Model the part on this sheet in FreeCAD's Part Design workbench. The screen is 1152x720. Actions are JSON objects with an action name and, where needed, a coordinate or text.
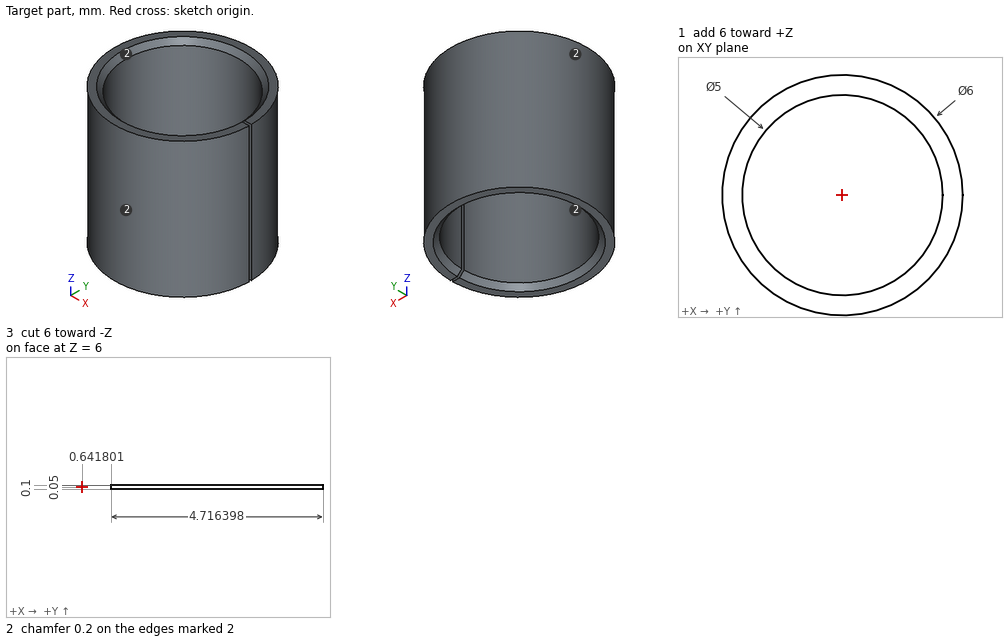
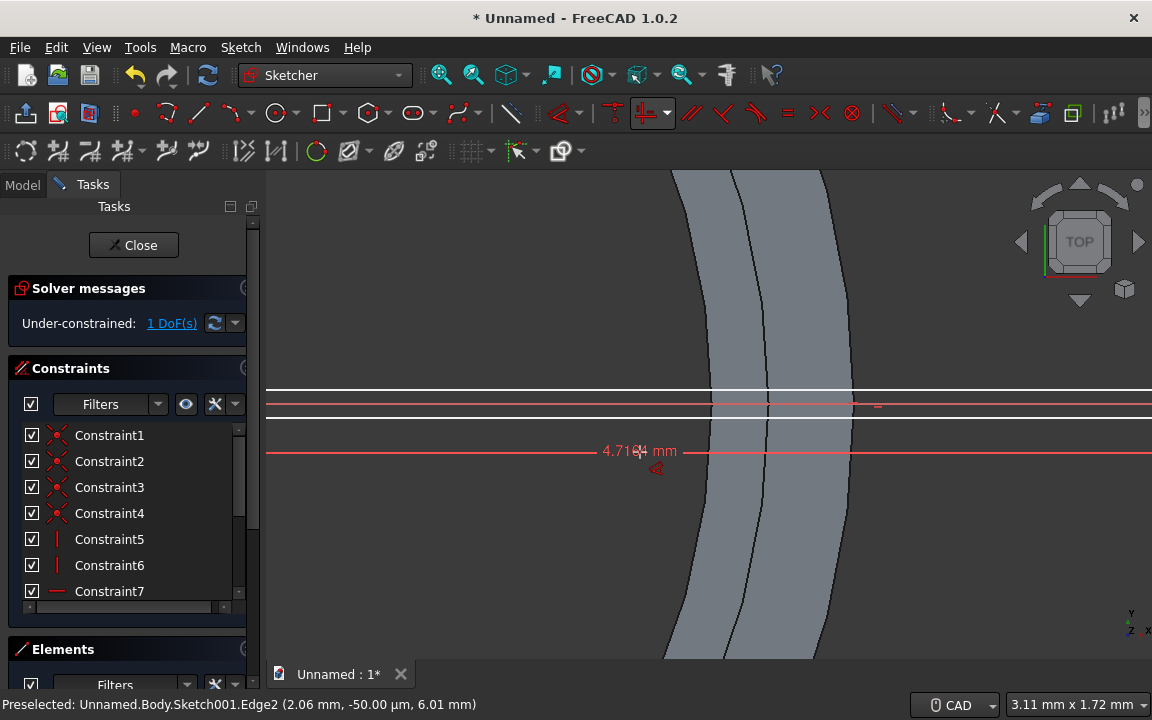
{"action": "scroll", "coordinate": [588, 419], "scroll_direction": "down", "scroll_amount": 6}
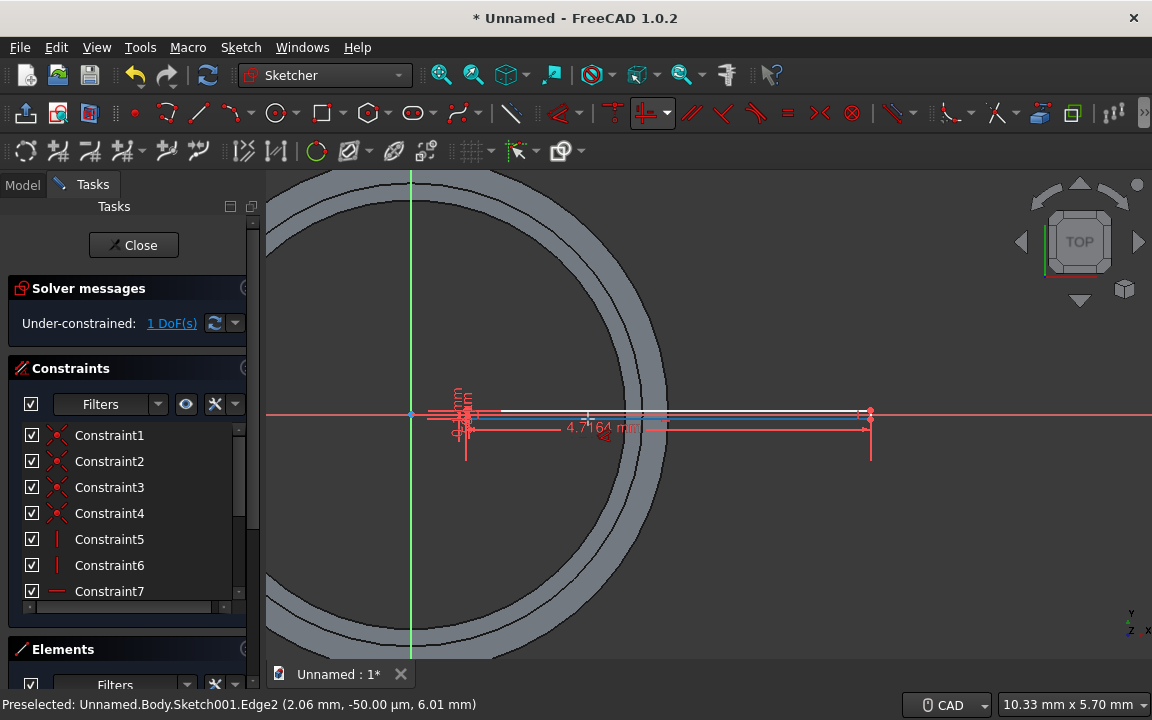
{"action": "scroll", "coordinate": [466, 411], "scroll_direction": "up", "scroll_amount": 2}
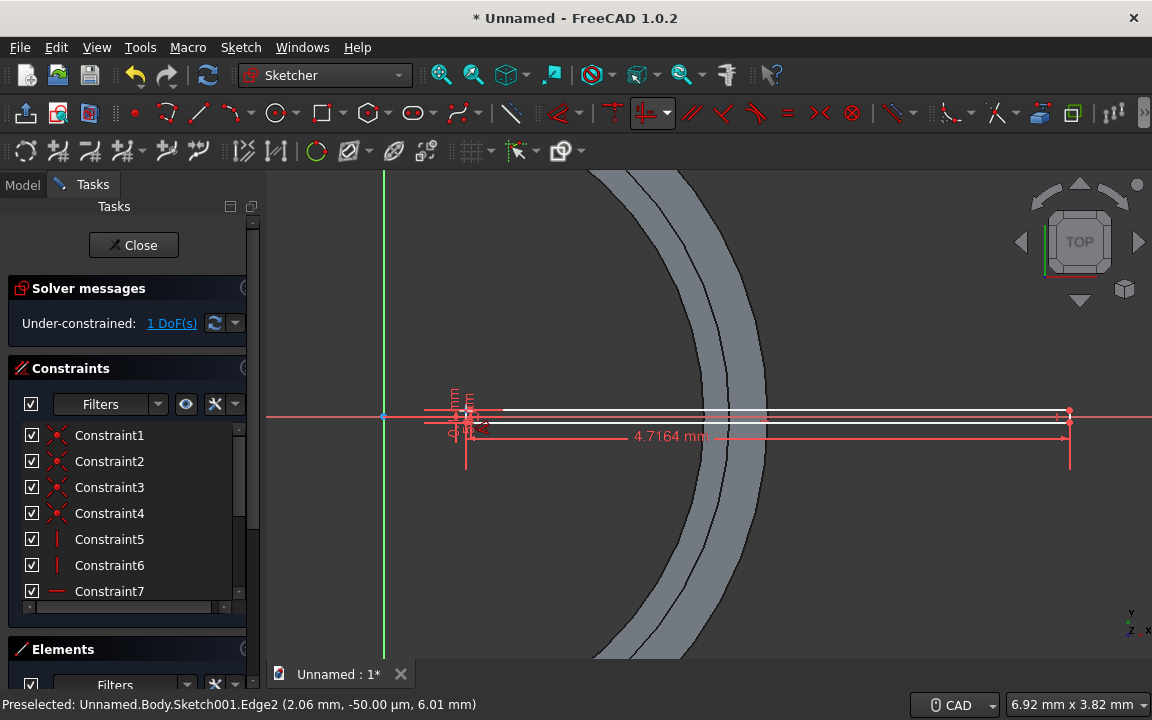
{"action": "left_click", "coordinate": [466, 410]}
{"action": "left_click", "coordinate": [425, 376]}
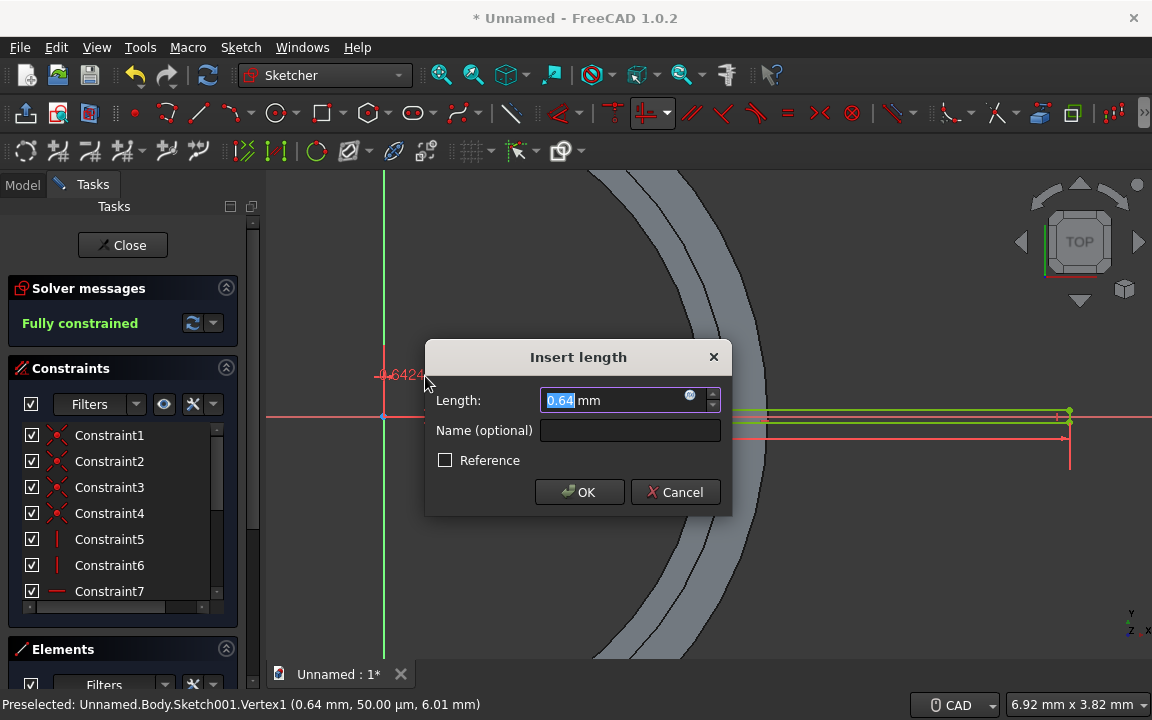
{"action": "type", "text": "0.641801"}
{"action": "key", "text": "Return"}
{"action": "key", "text": "Escape"}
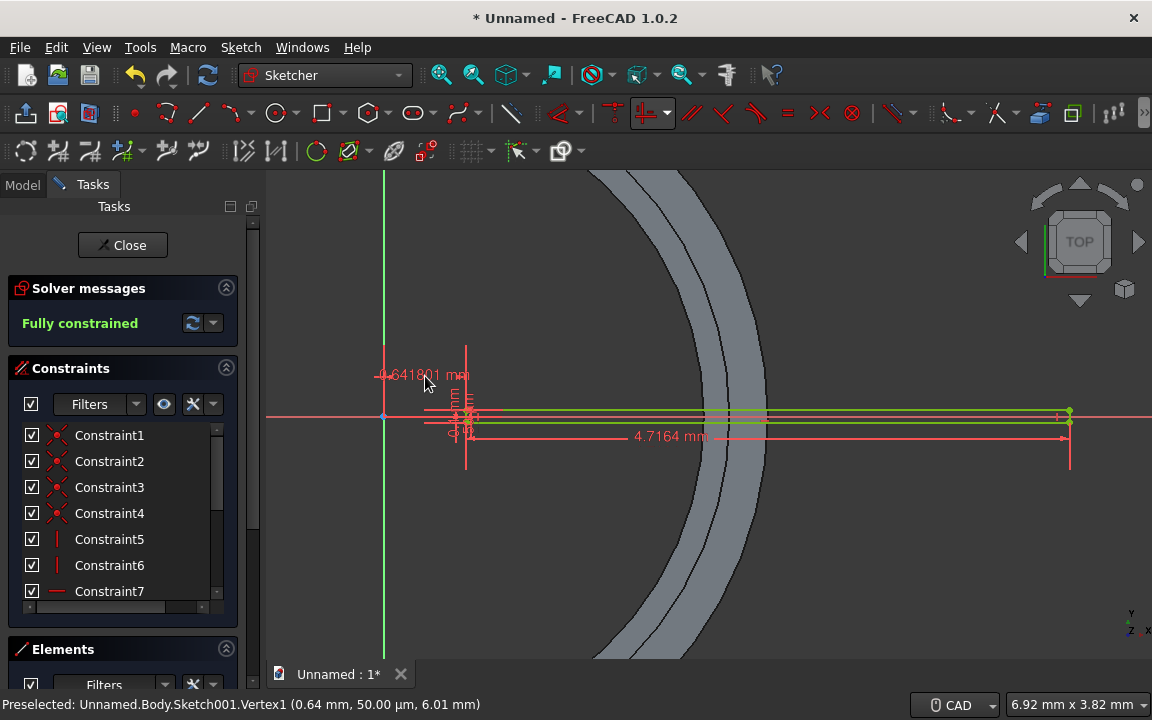
{"action": "left_click", "coordinate": [123, 245]}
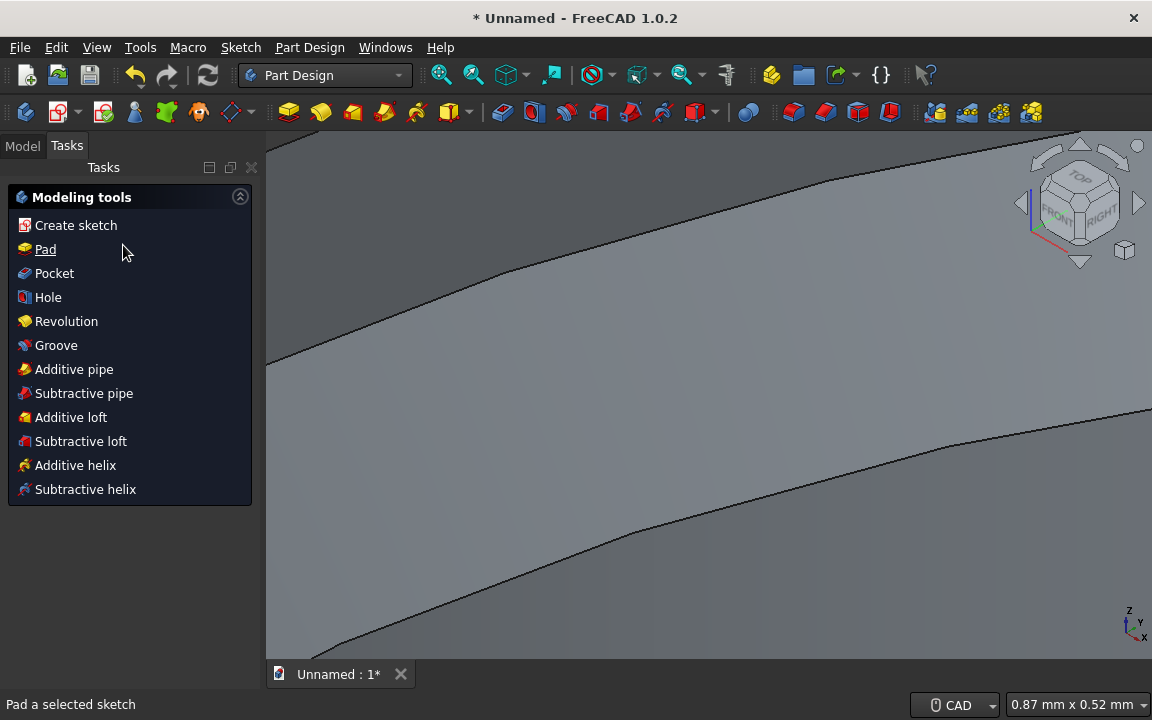
{"action": "left_click", "coordinate": [504, 112]}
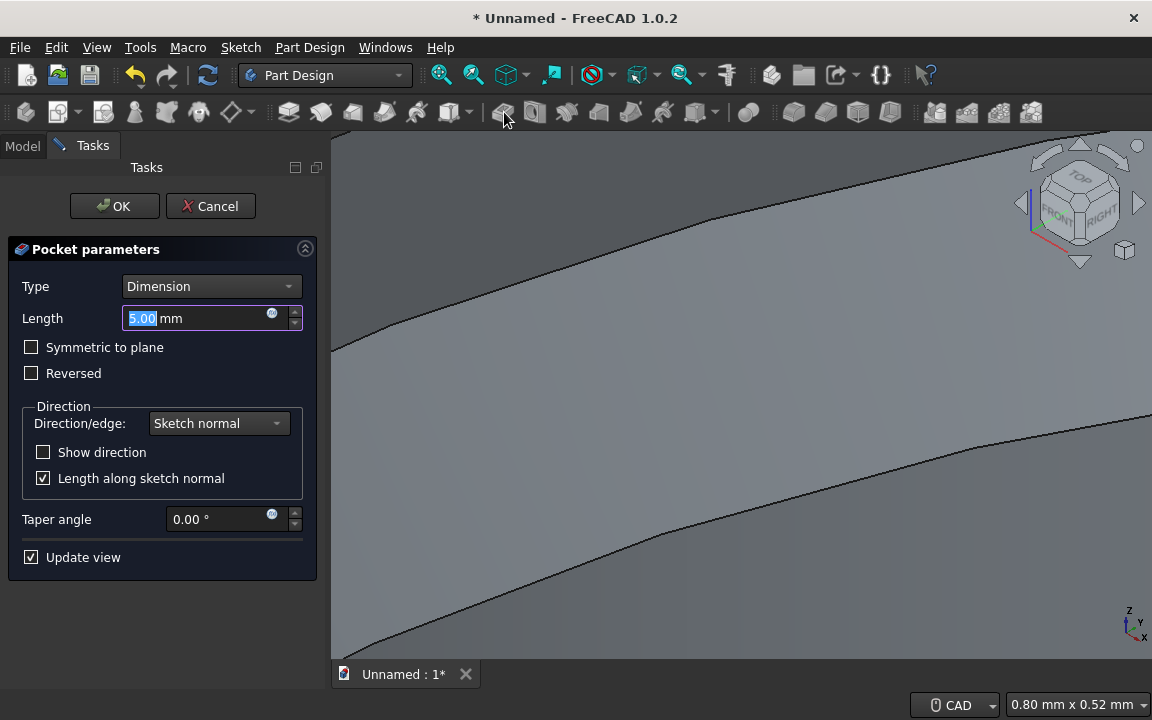
{"action": "type", "text": "6"}
{"action": "key", "text": "Tab"}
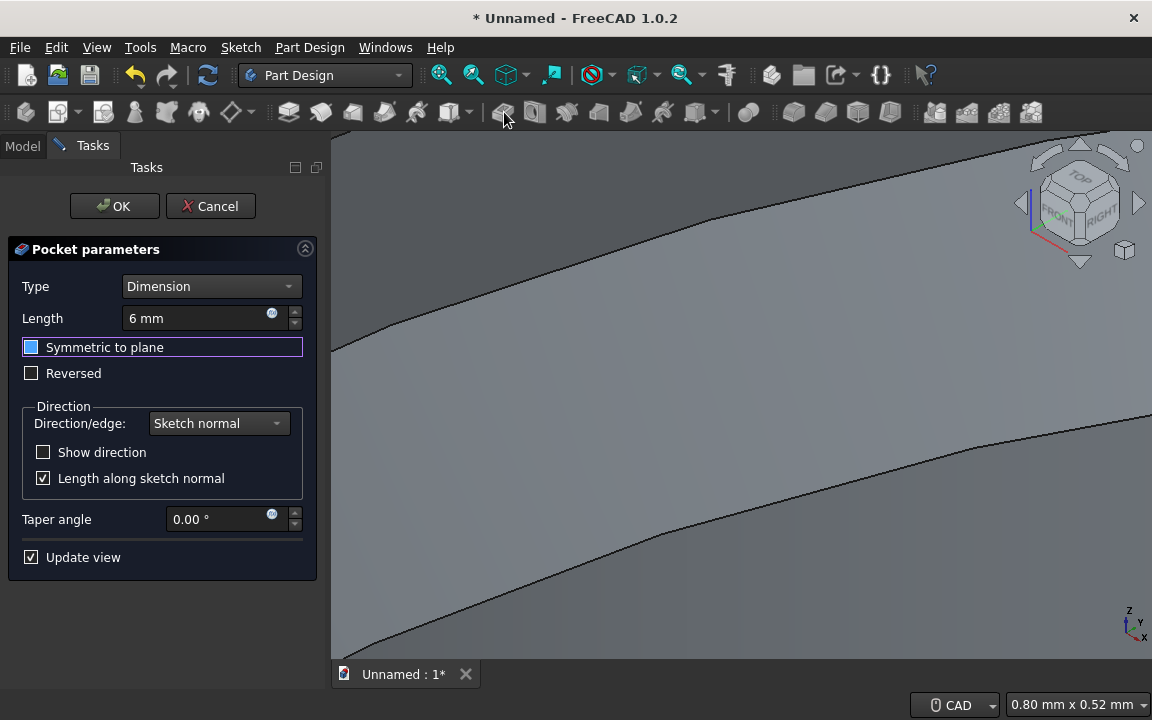
{"action": "left_click", "coordinate": [115, 206]}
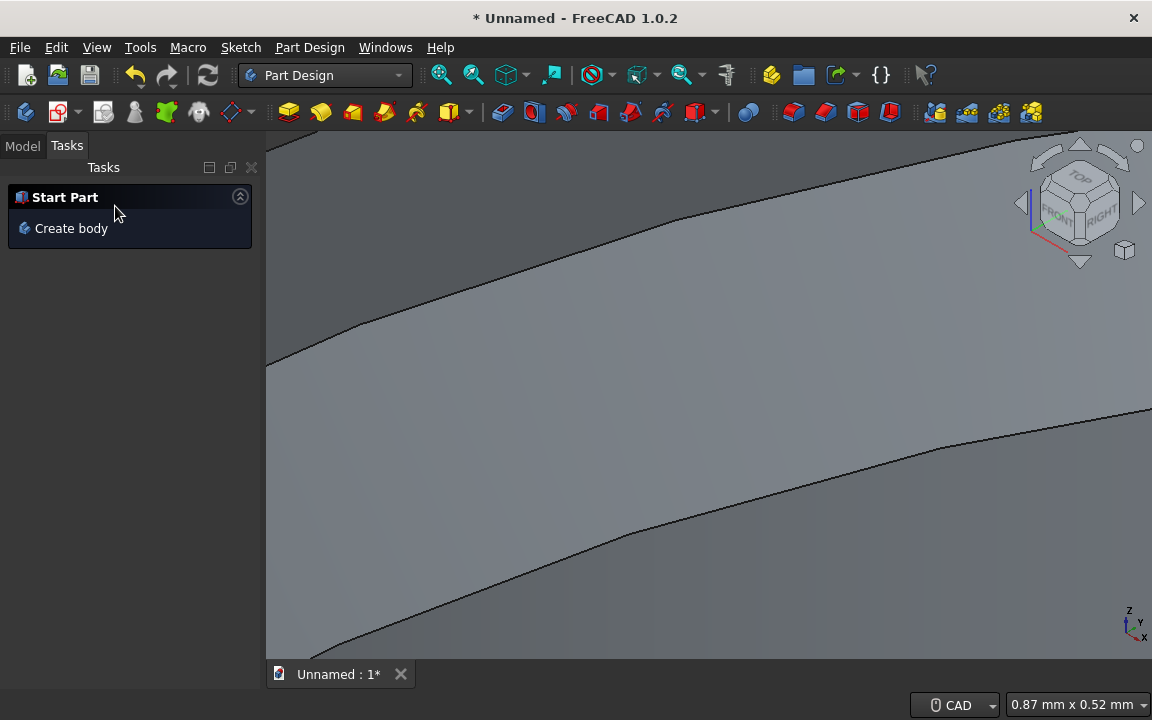
{"action": "left_click", "coordinate": [442, 76]}